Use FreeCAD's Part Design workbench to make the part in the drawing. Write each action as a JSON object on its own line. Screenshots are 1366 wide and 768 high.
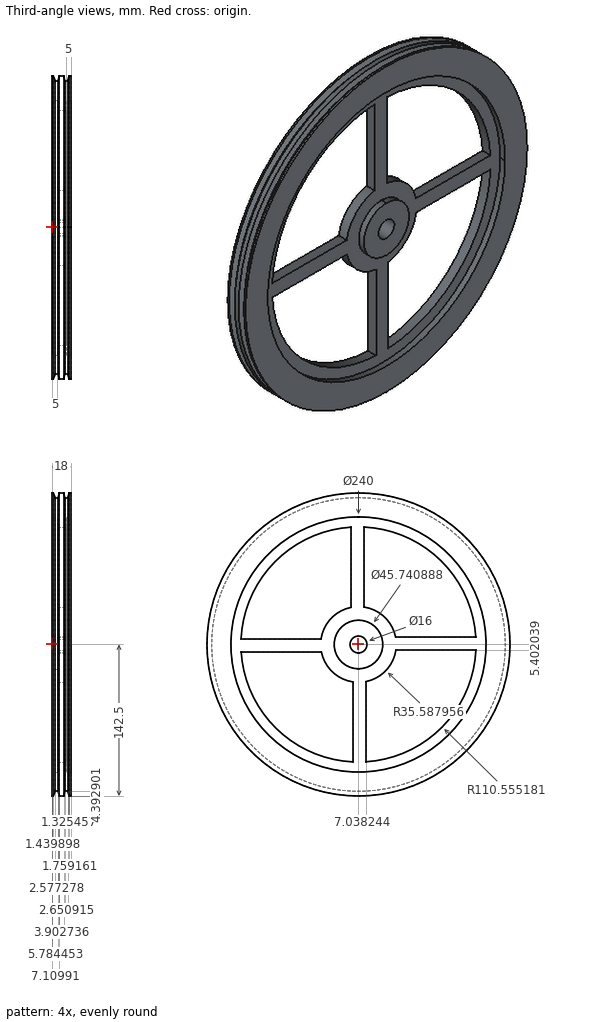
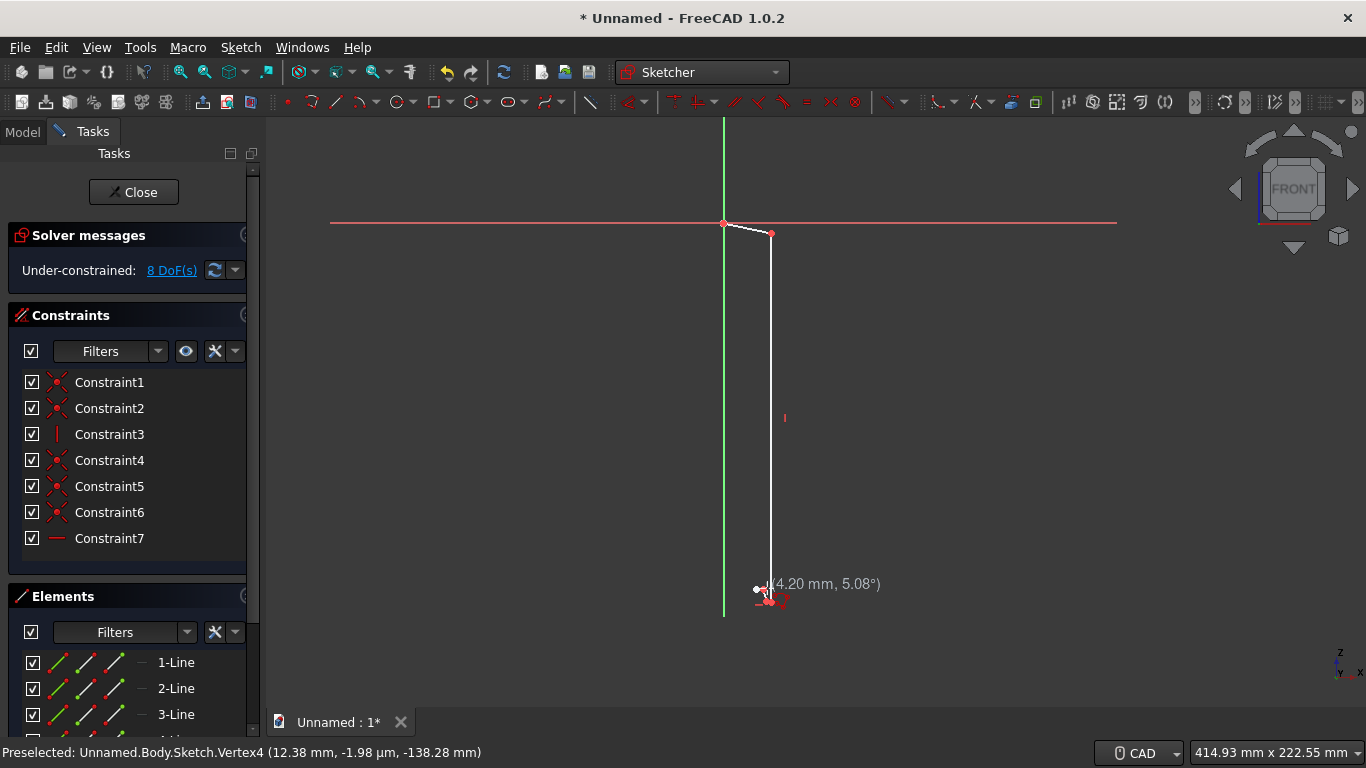
{"action": "scroll", "coordinate": [753, 601], "scroll_direction": "up", "scroll_amount": 2}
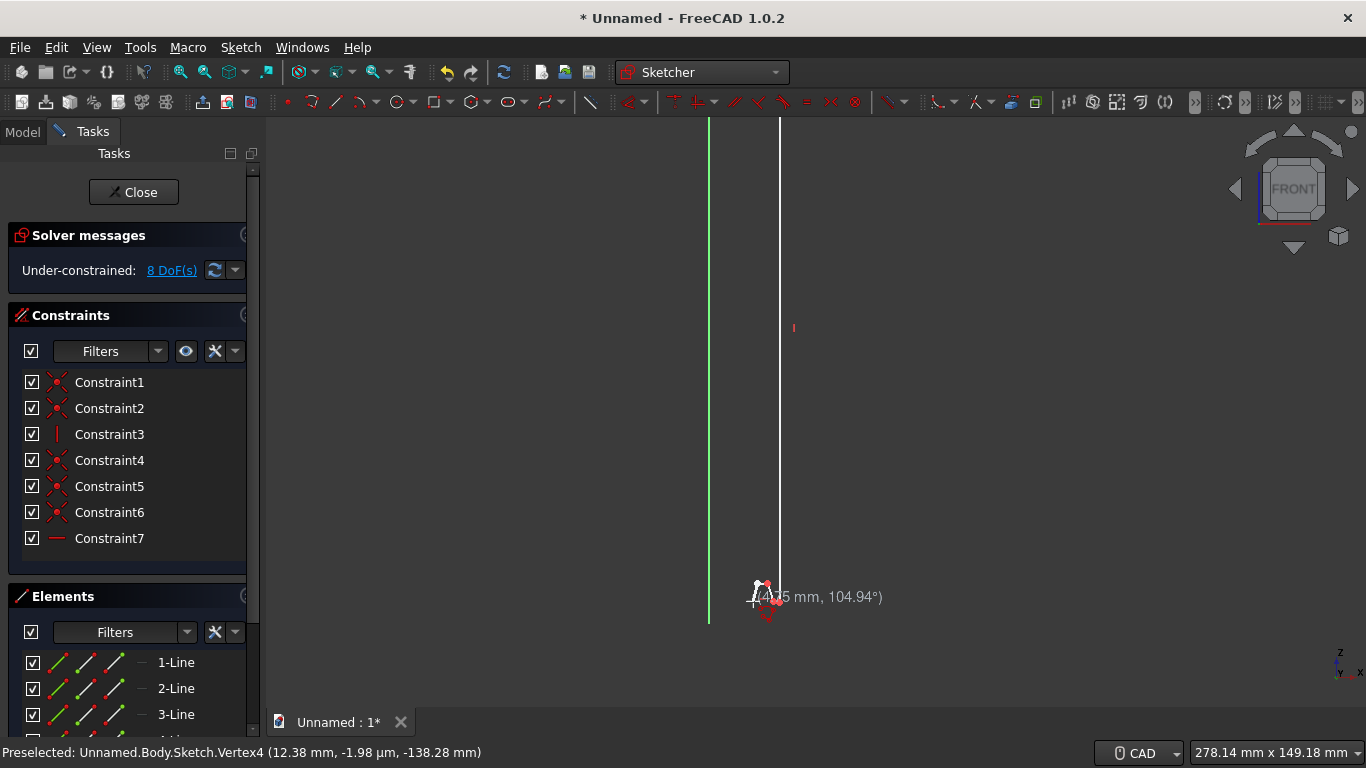
{"action": "left_click", "coordinate": [753, 601]}
{"action": "left_click", "coordinate": [737, 601]}
{"action": "left_click", "coordinate": [732, 584]}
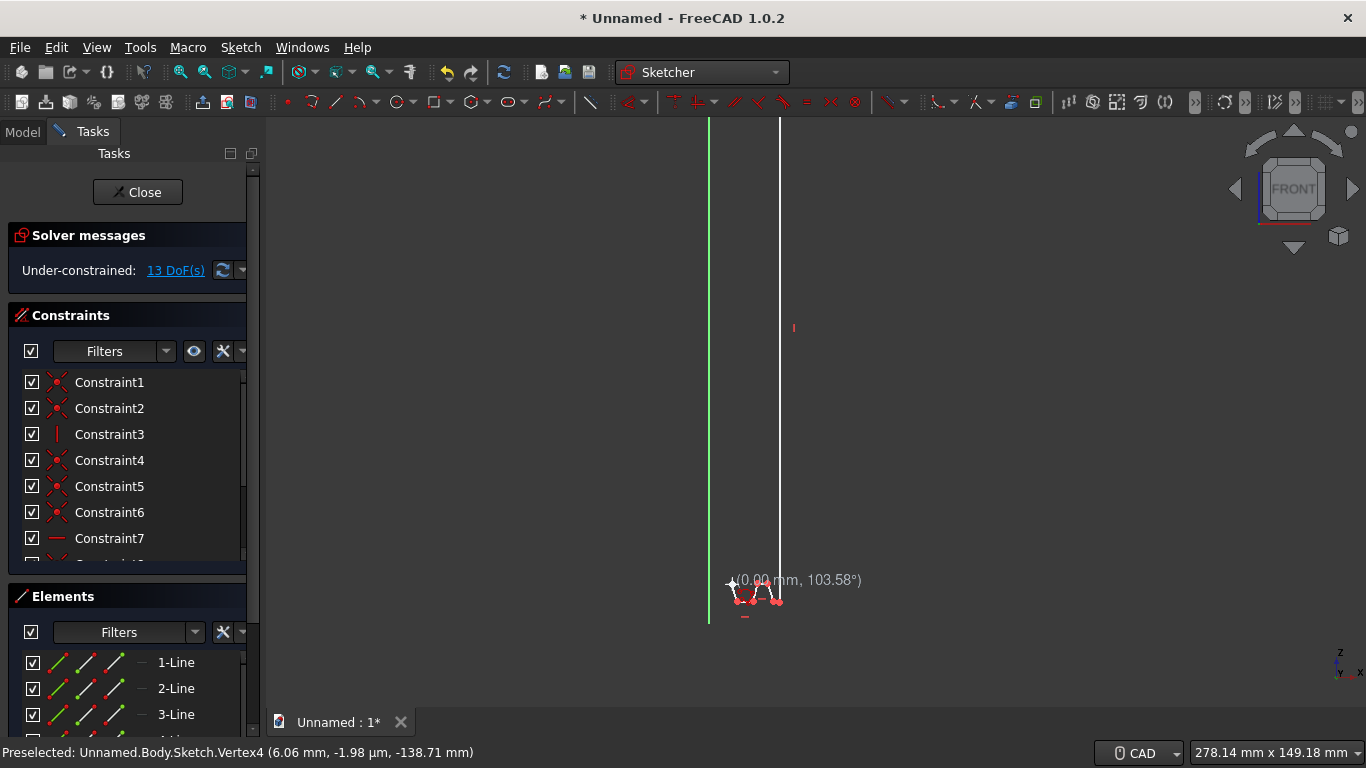
{"action": "scroll", "coordinate": [722, 584], "scroll_direction": "up", "scroll_amount": 3}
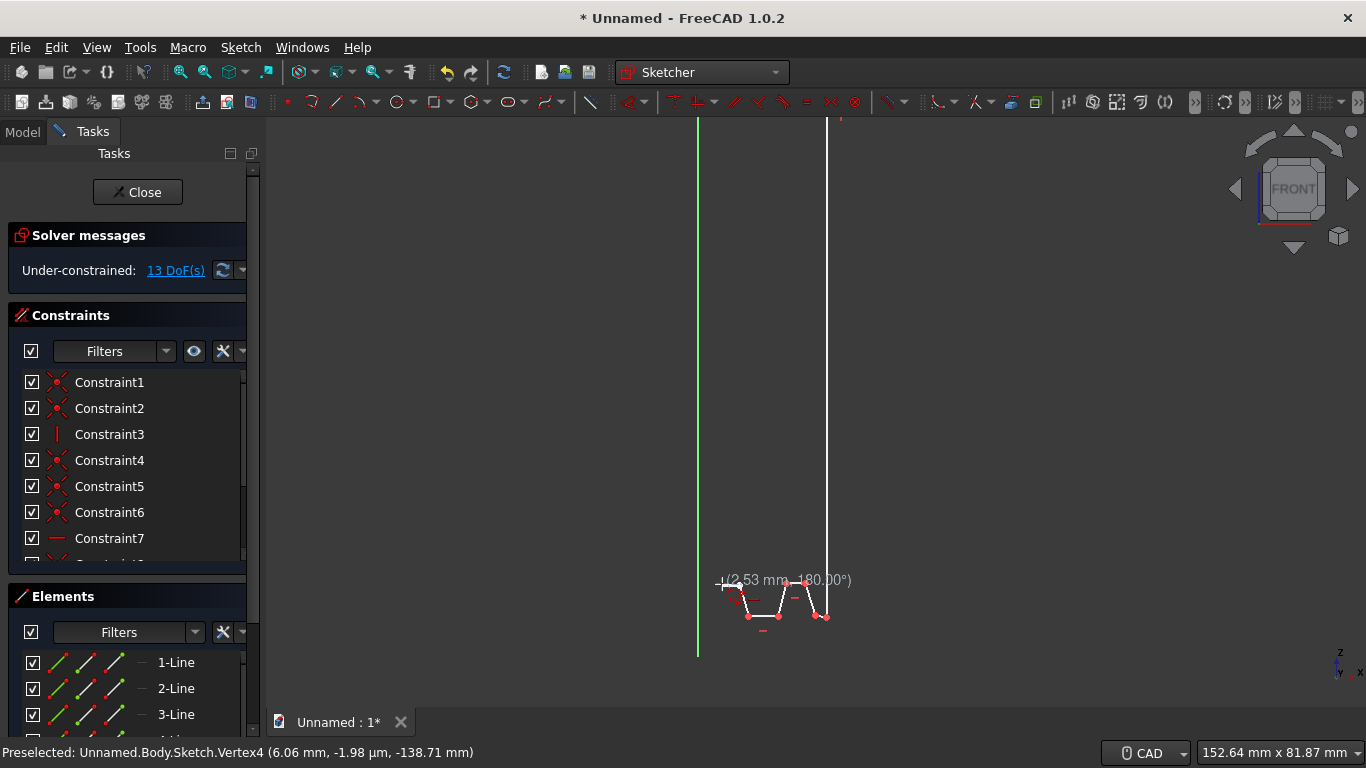
{"action": "left_click", "coordinate": [721, 583]}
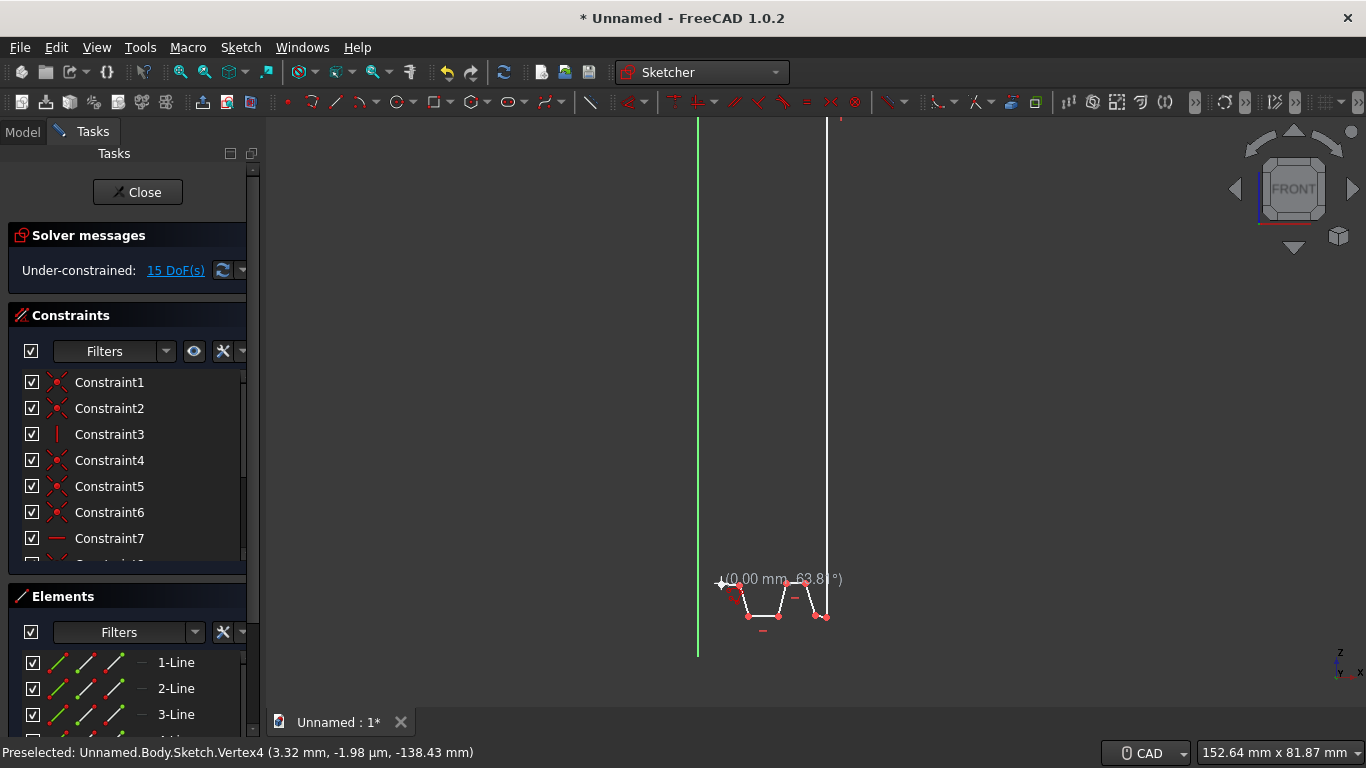
{"action": "scroll", "coordinate": [708, 614], "scroll_direction": "up", "scroll_amount": 3}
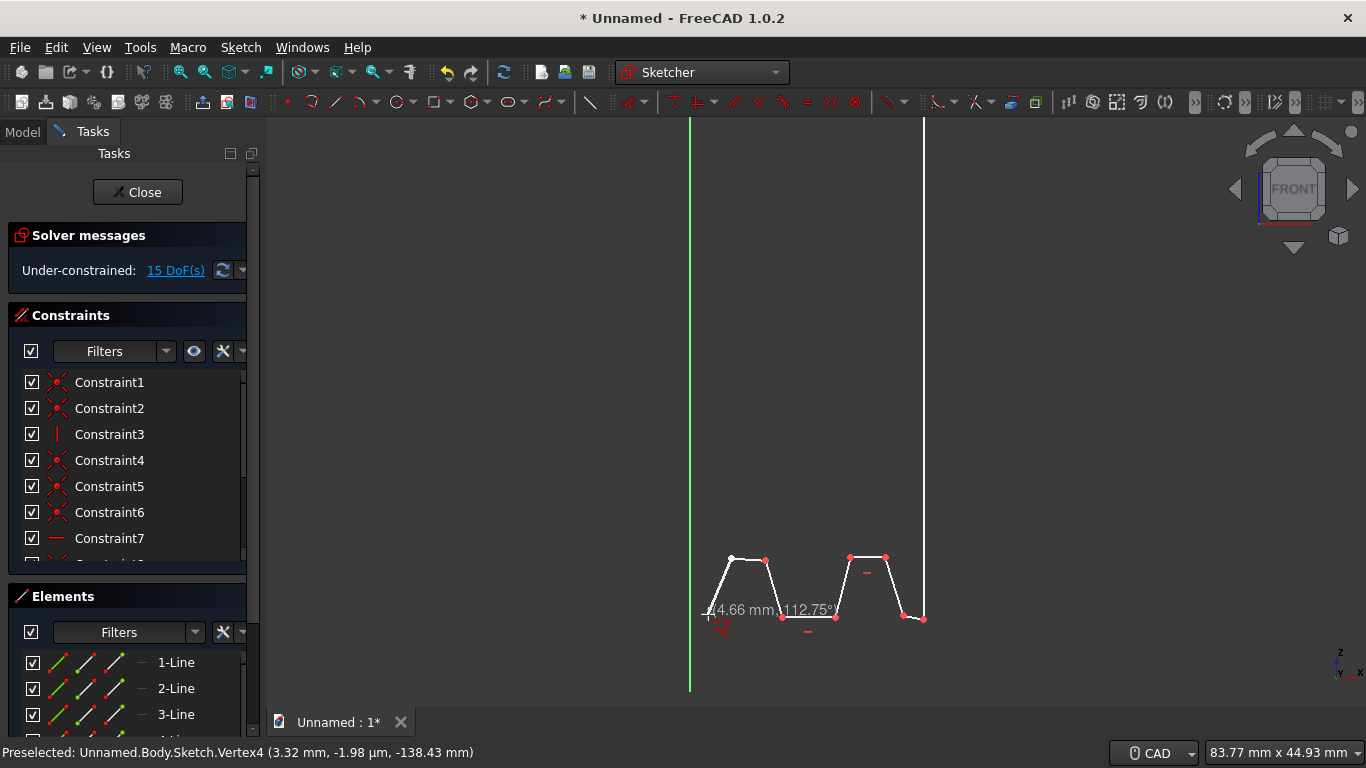
{"action": "left_click", "coordinate": [708, 614]}
{"action": "left_click", "coordinate": [699, 614]}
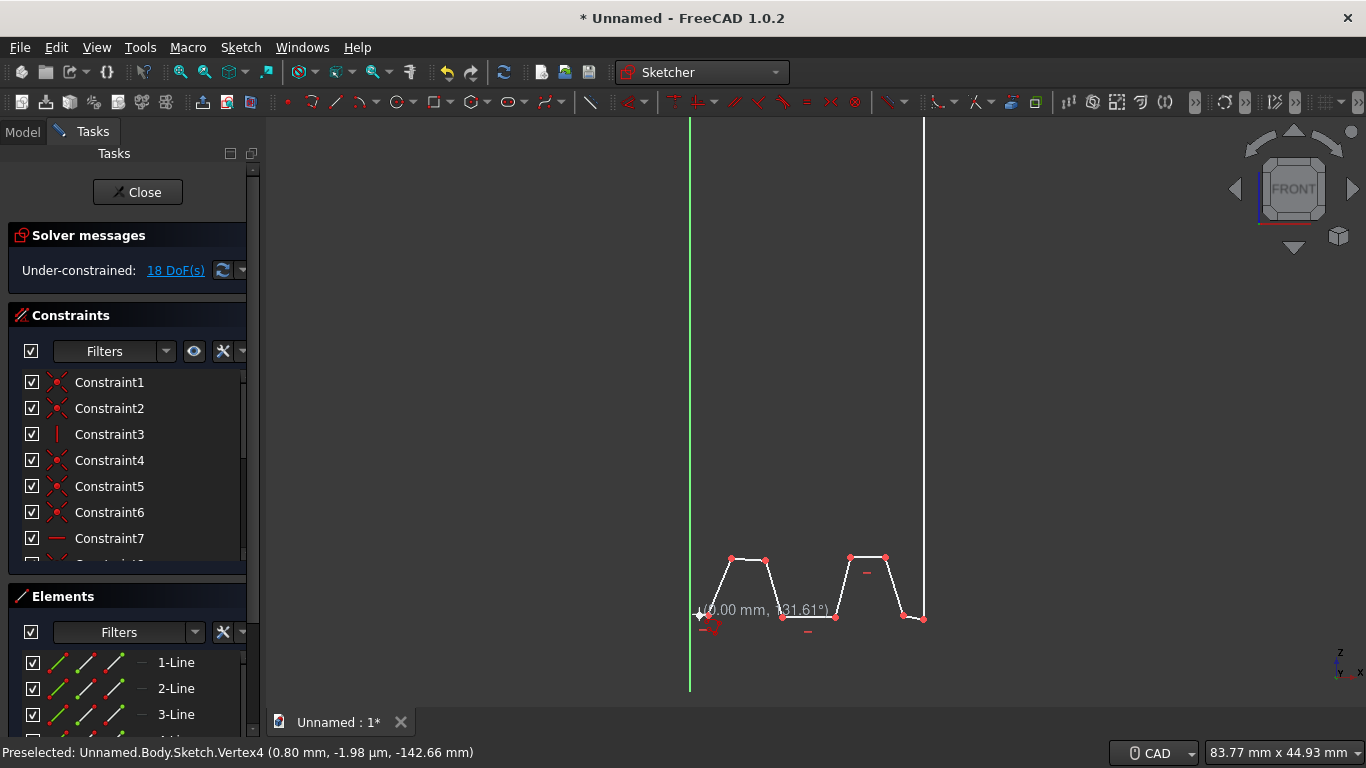
{"action": "scroll", "coordinate": [732, 598], "scroll_direction": "down", "scroll_amount": 8}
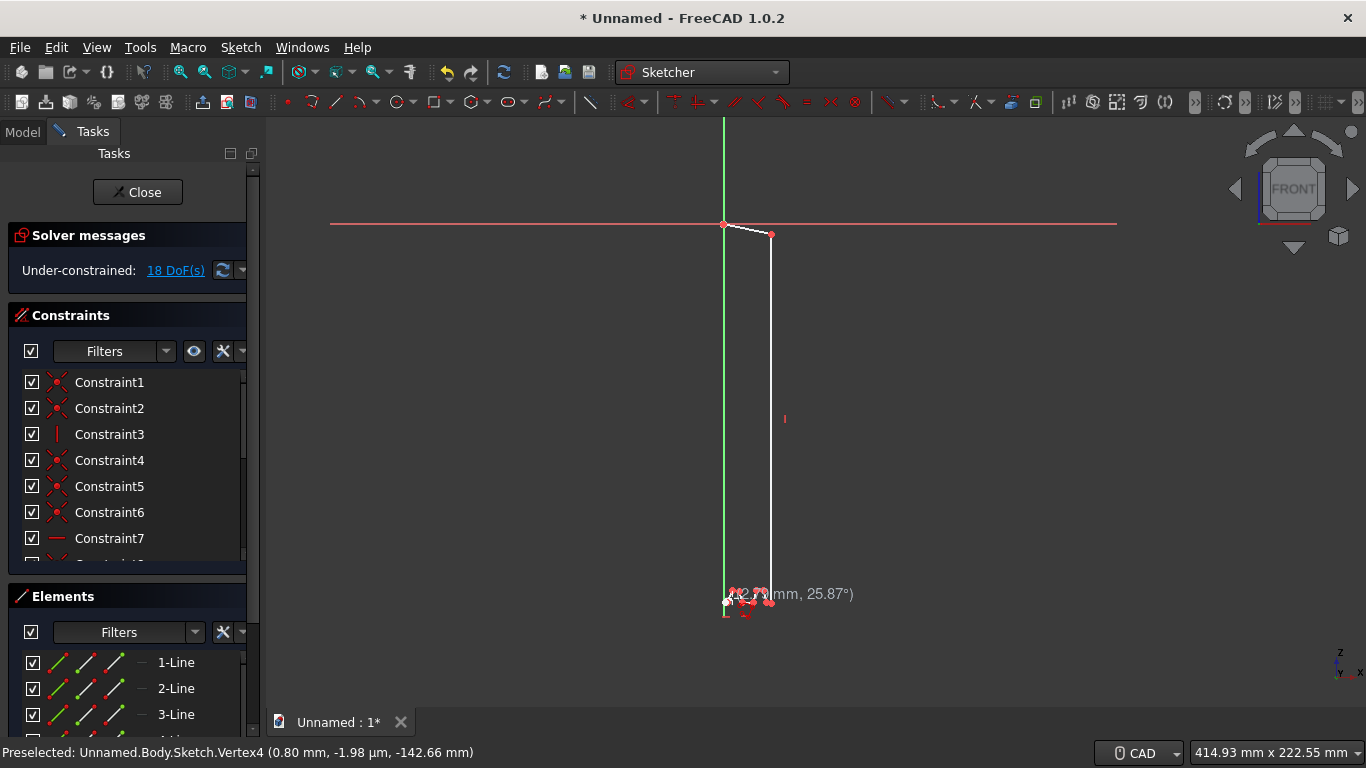
{"action": "left_click", "coordinate": [724, 224]}
{"action": "key", "text": "Escape"}
{"action": "key", "text": "Escape"}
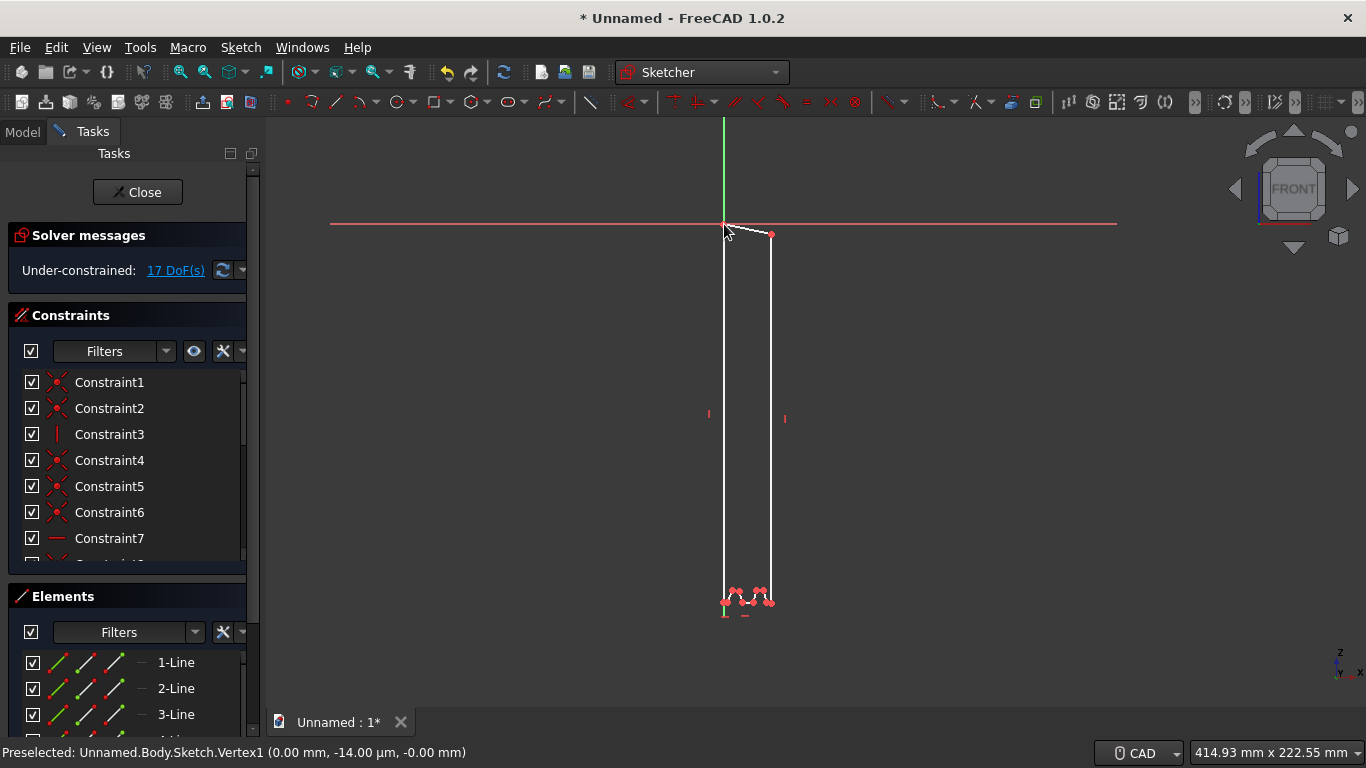
{"action": "left_click", "coordinate": [738, 227]}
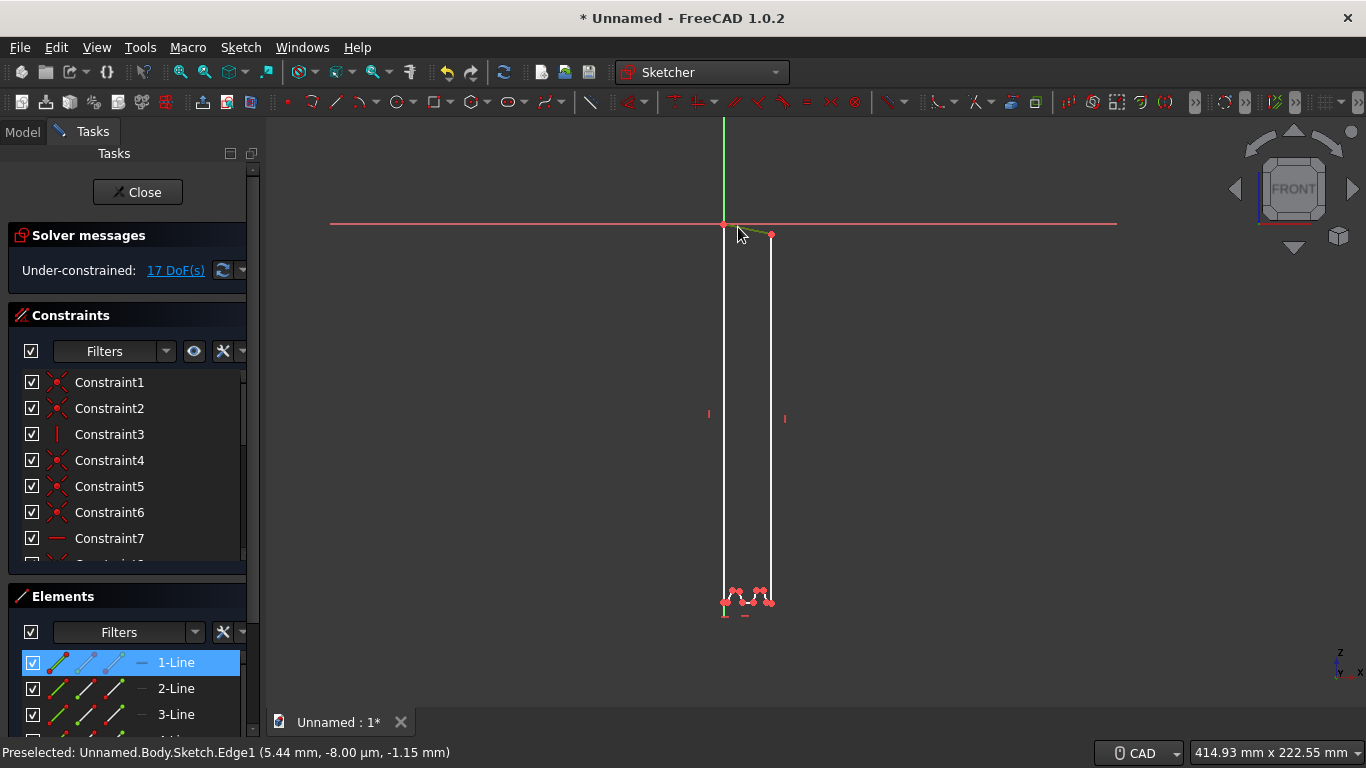
{"action": "key", "text": "h"}